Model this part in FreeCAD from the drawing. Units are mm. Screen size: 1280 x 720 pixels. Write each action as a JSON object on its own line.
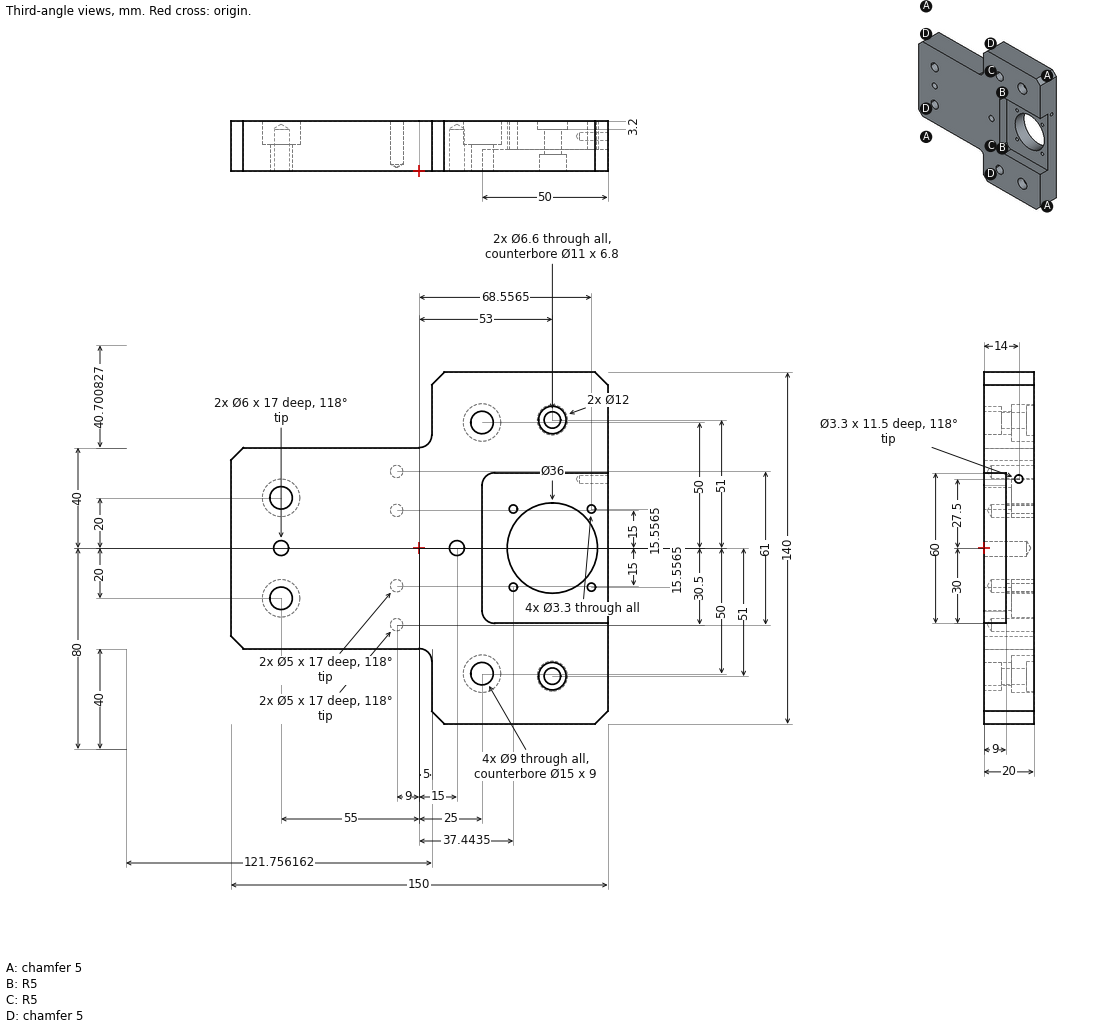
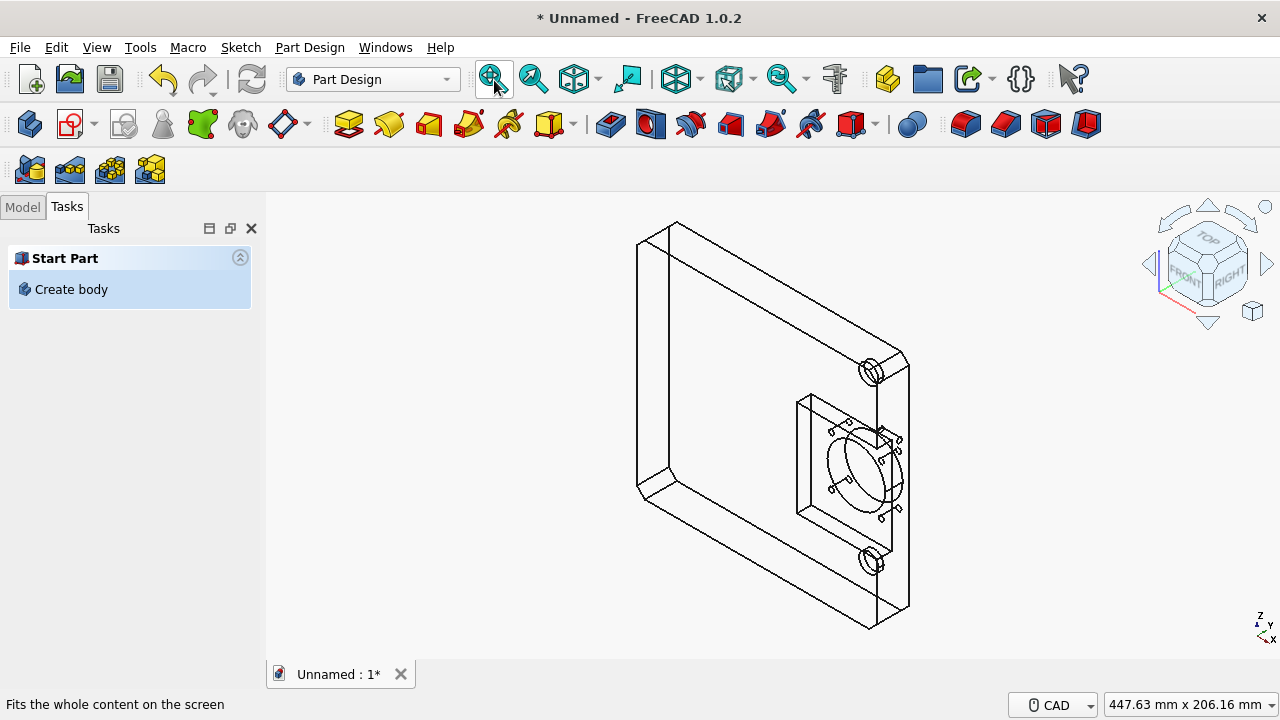
{"action": "left_click", "coordinate": [804, 397]}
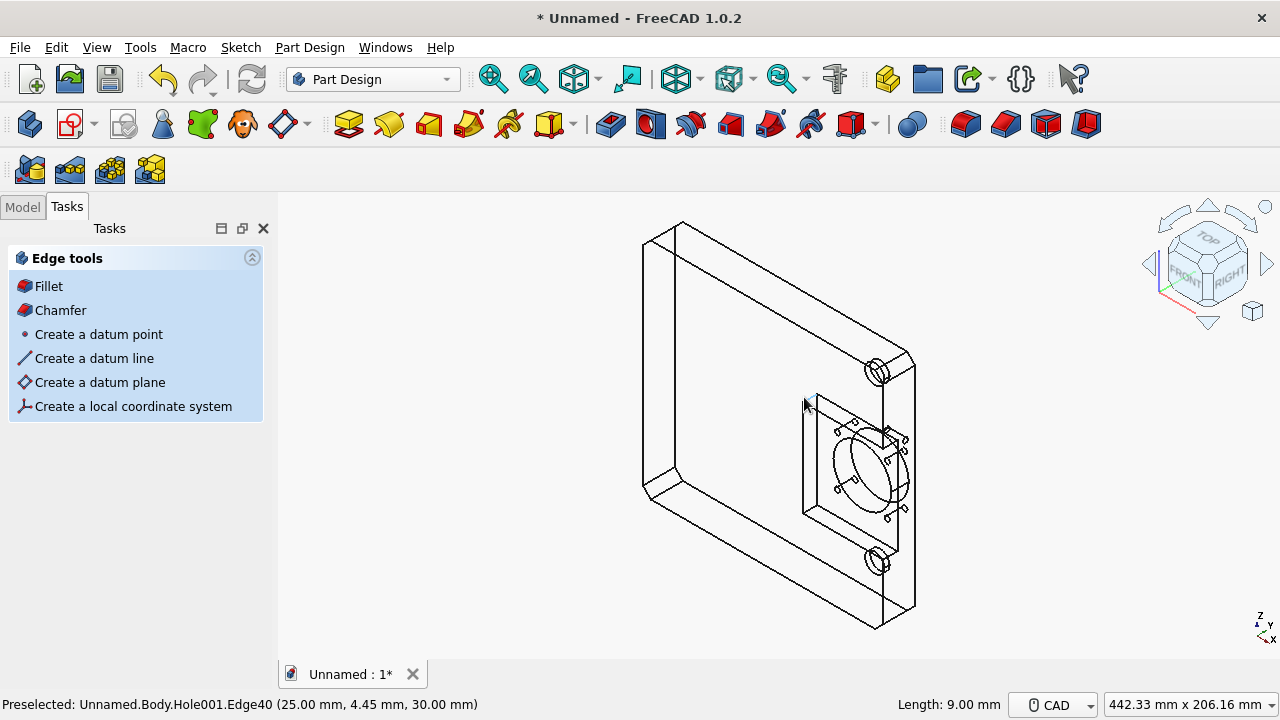
{"action": "left_click", "coordinate": [810, 508], "text": "ctrl"}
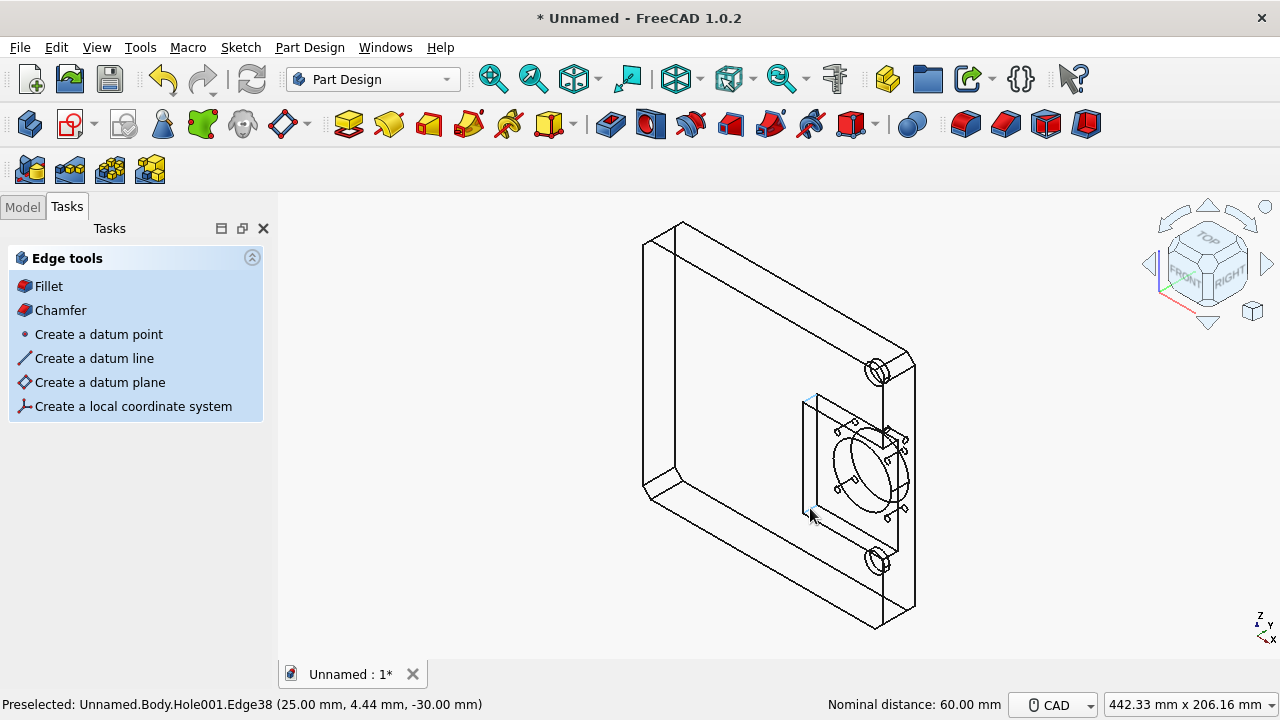
{"action": "key", "text": "v 1"}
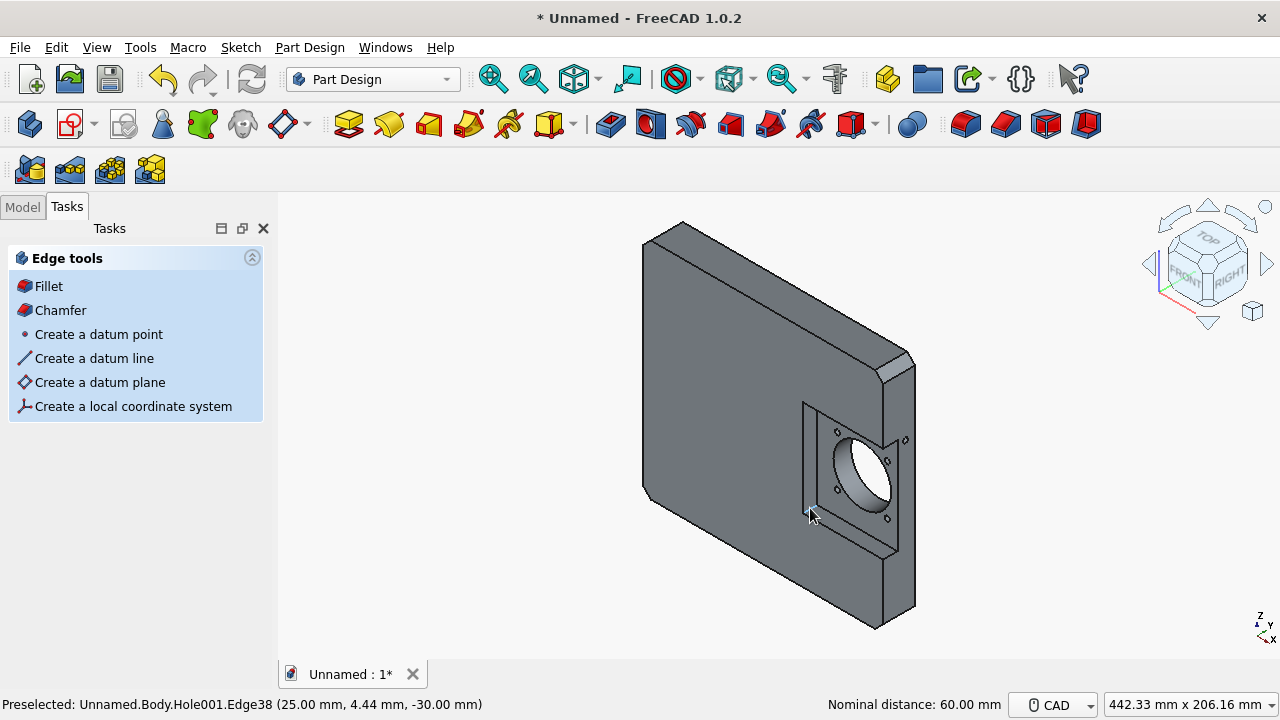
{"action": "left_click", "coordinate": [966, 124]}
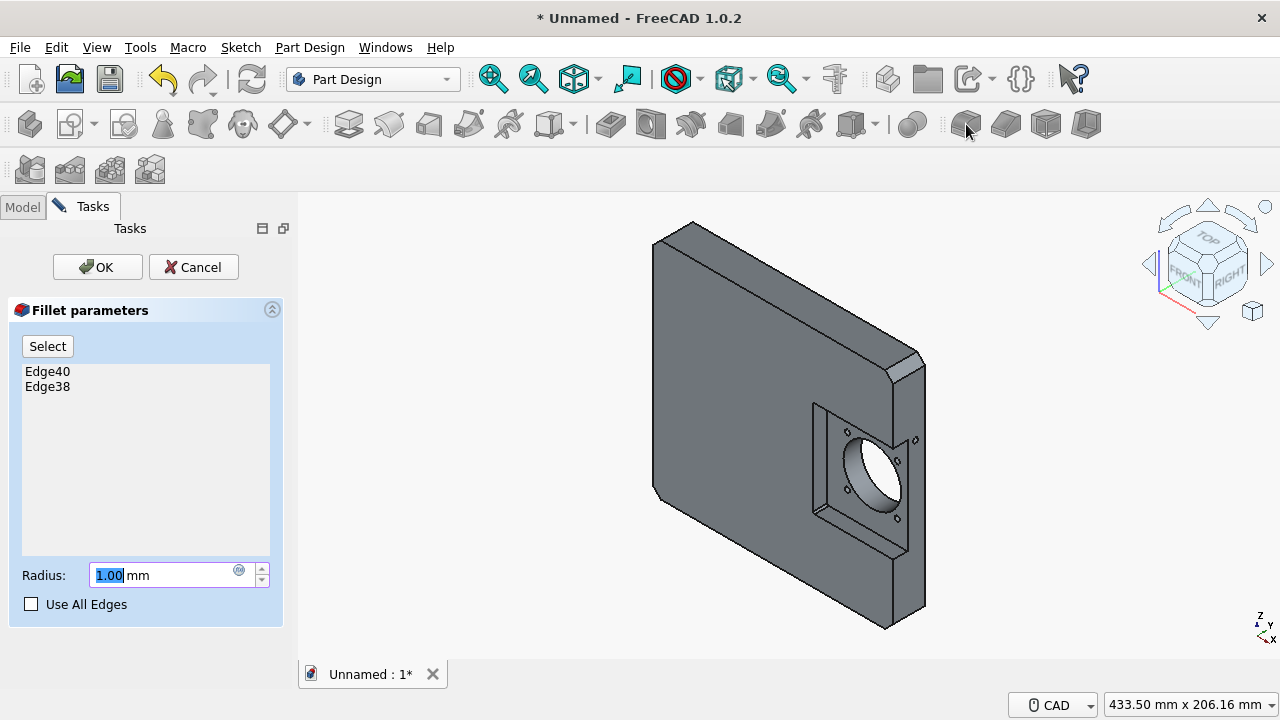
{"action": "type", "text": "5"}
{"action": "key", "text": "Tab"}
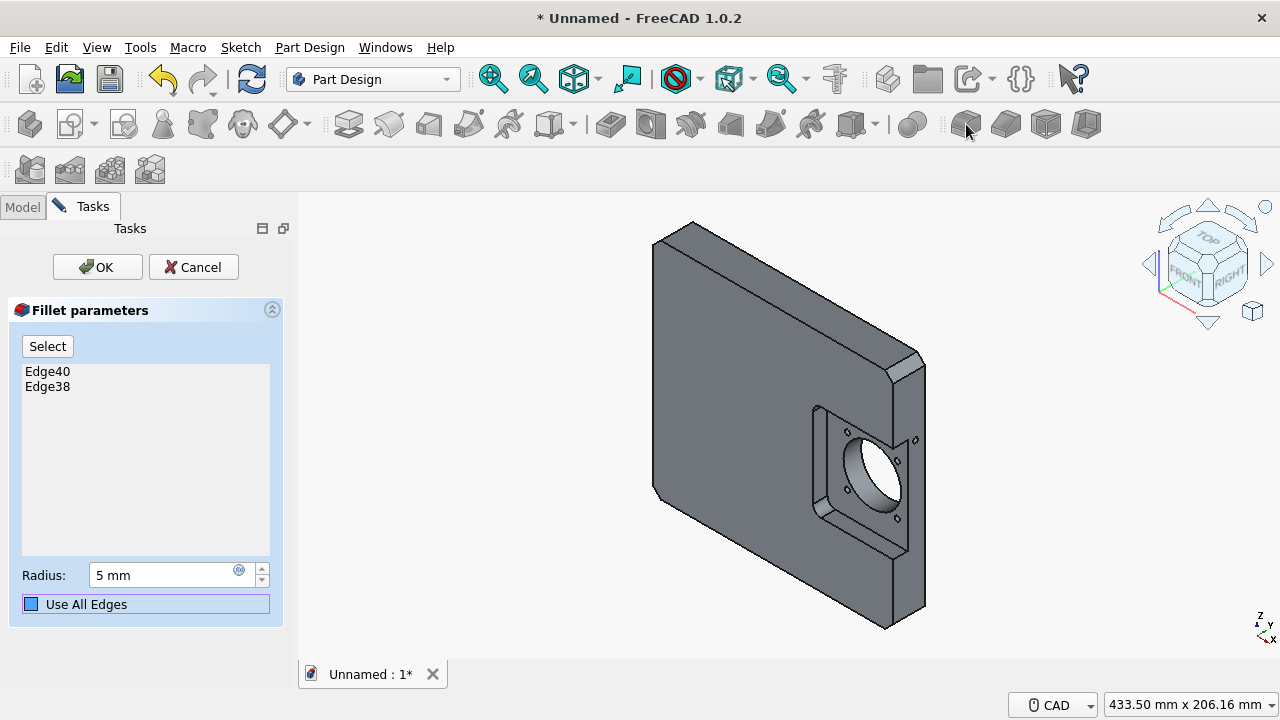
{"action": "left_click", "coordinate": [98, 267]}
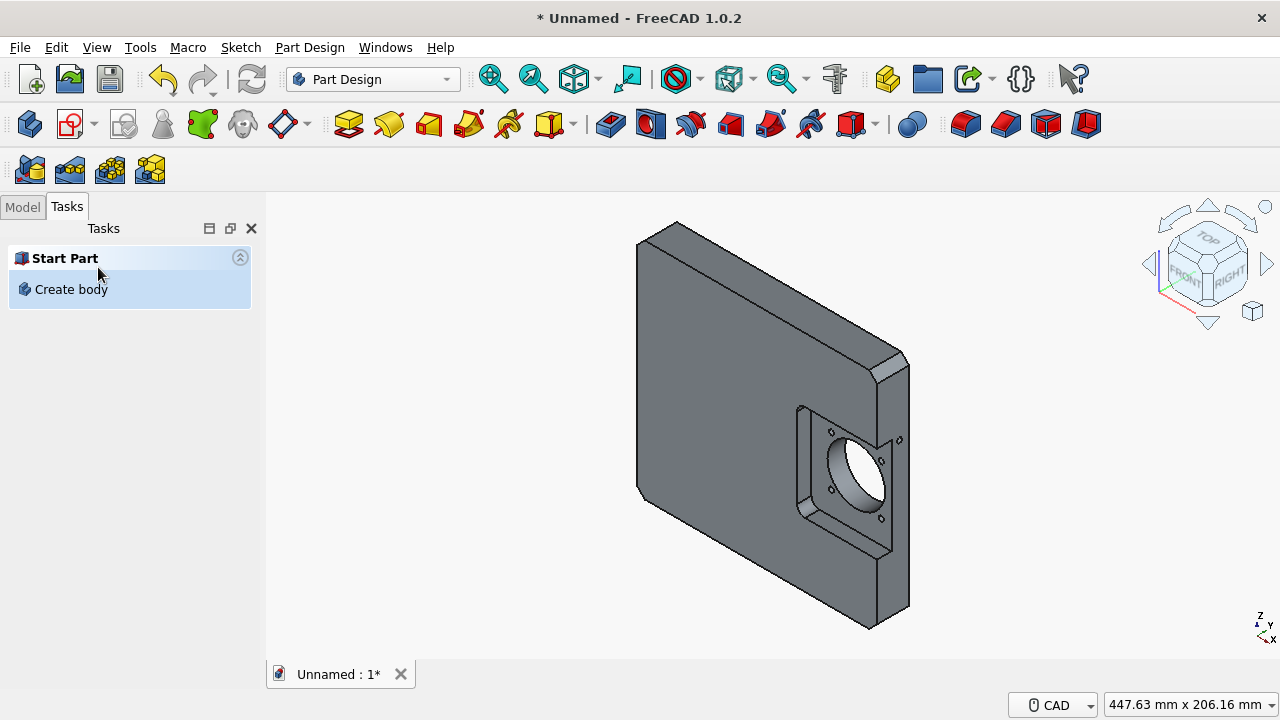
{"action": "left_click", "coordinate": [70, 124]}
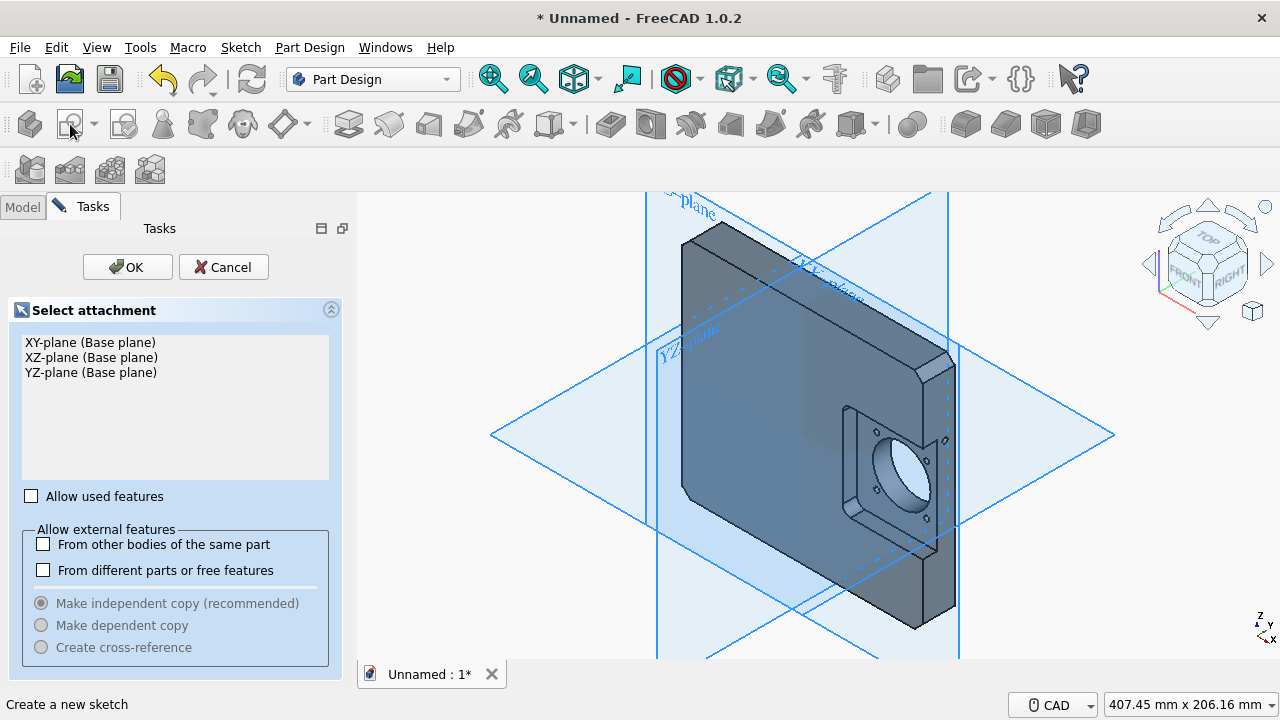
{"action": "left_click", "coordinate": [82, 358]}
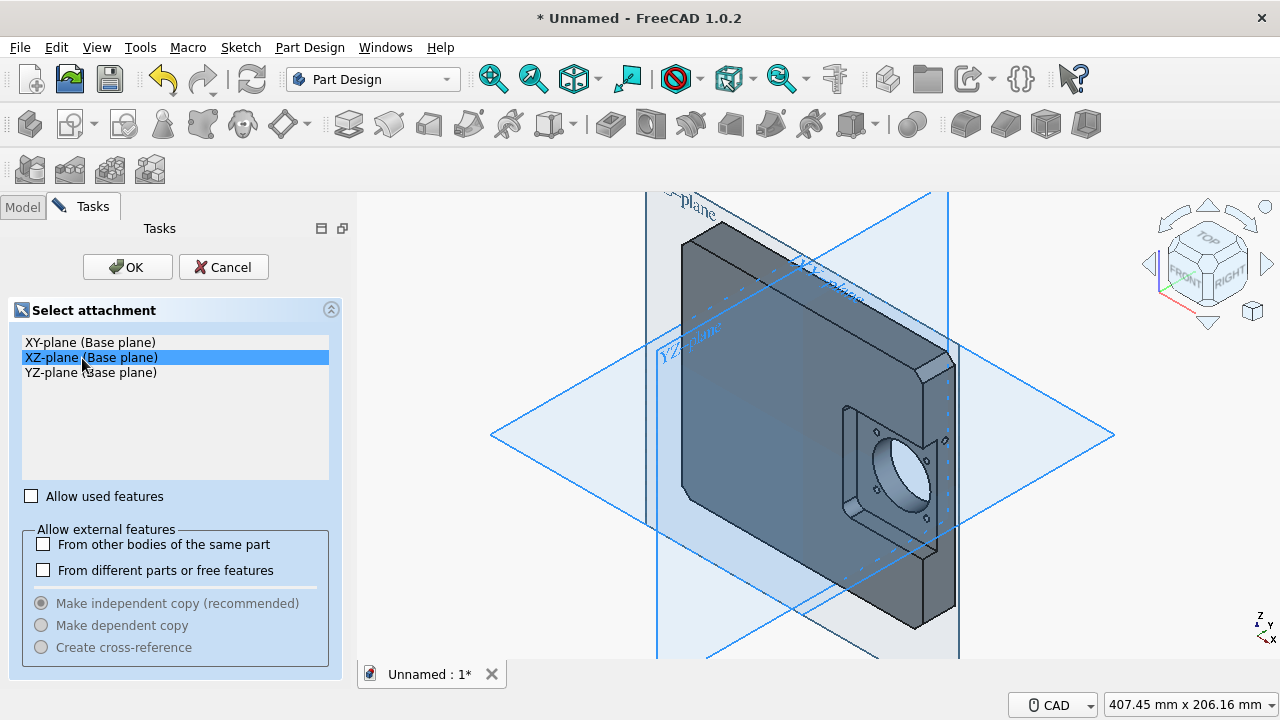
{"action": "left_click", "coordinate": [128, 267]}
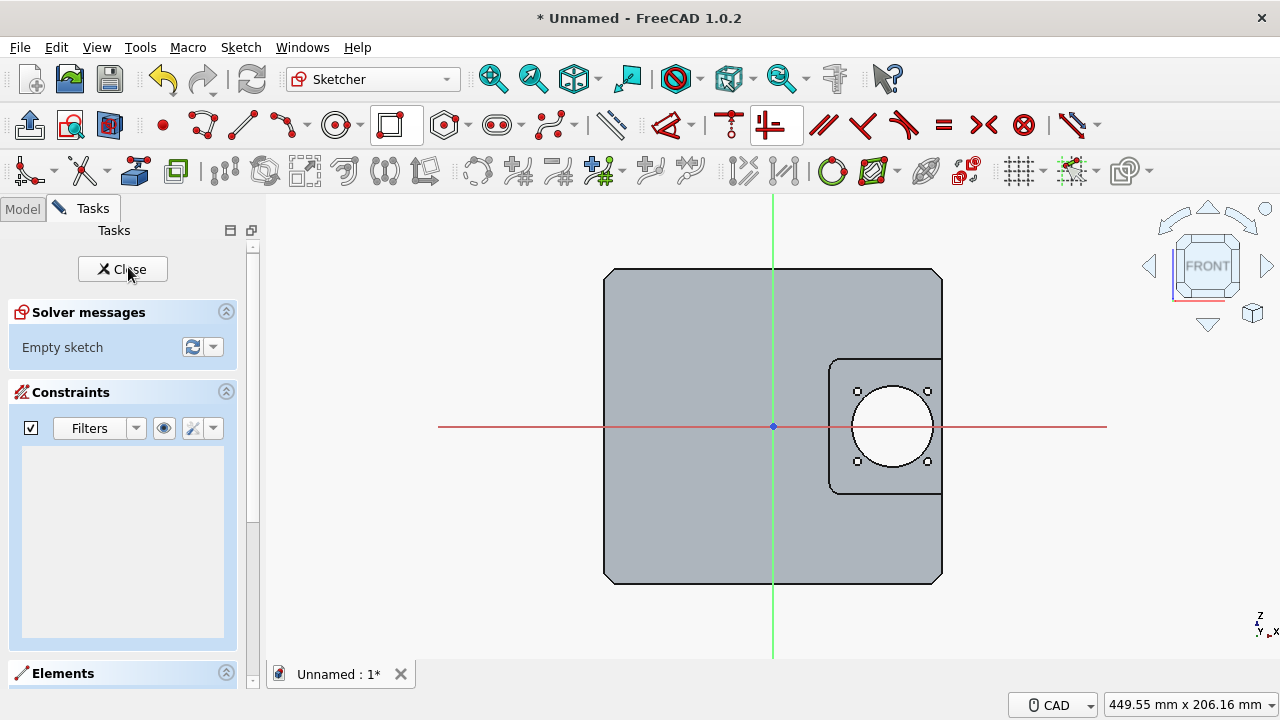
{"action": "left_click", "coordinate": [336, 126]}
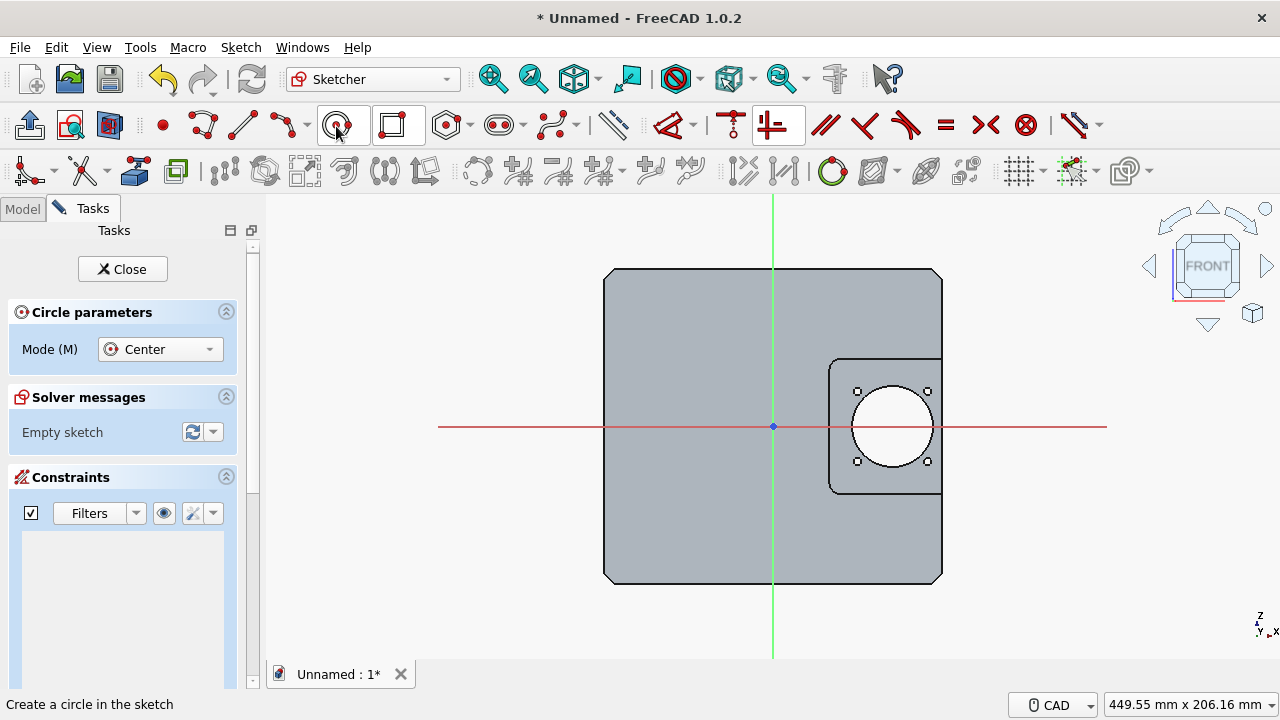
{"action": "scroll", "coordinate": [893, 311], "scroll_direction": "up", "scroll_amount": 6}